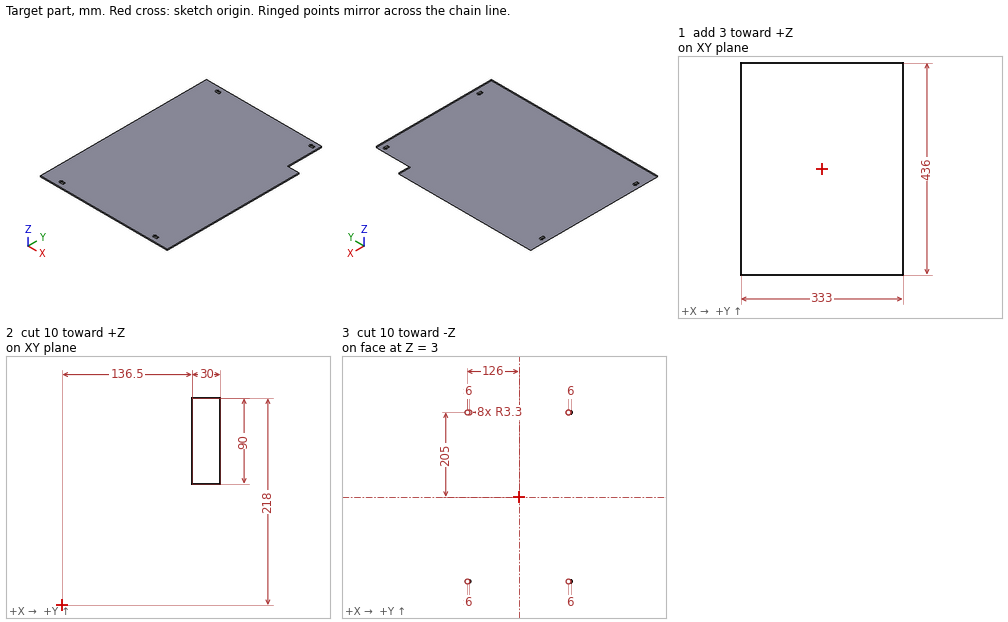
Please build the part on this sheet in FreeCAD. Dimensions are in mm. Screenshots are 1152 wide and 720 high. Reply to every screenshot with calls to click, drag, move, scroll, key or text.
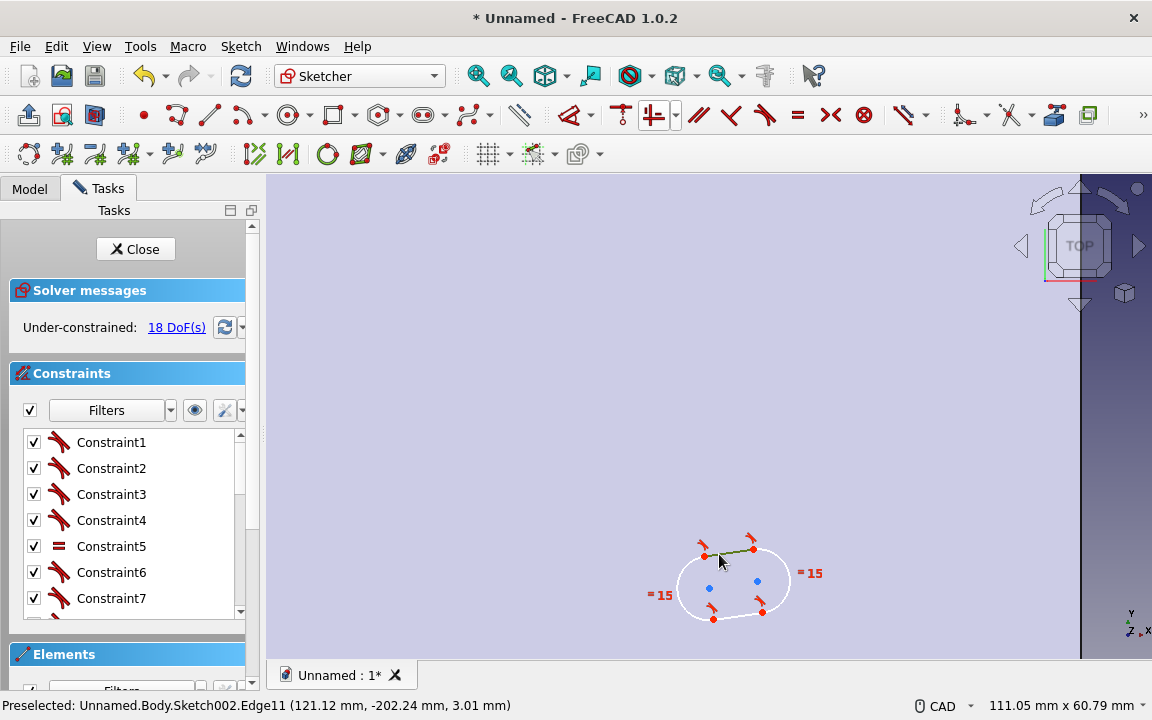
key(h)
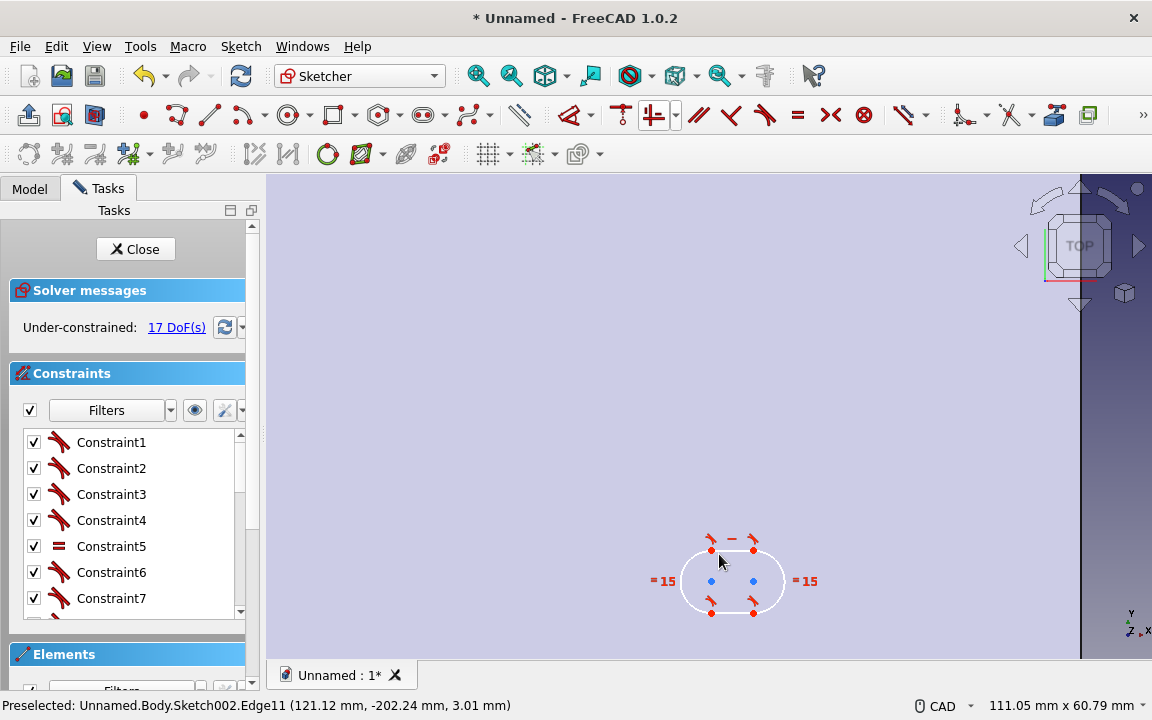
scroll(729, 564, down, 12)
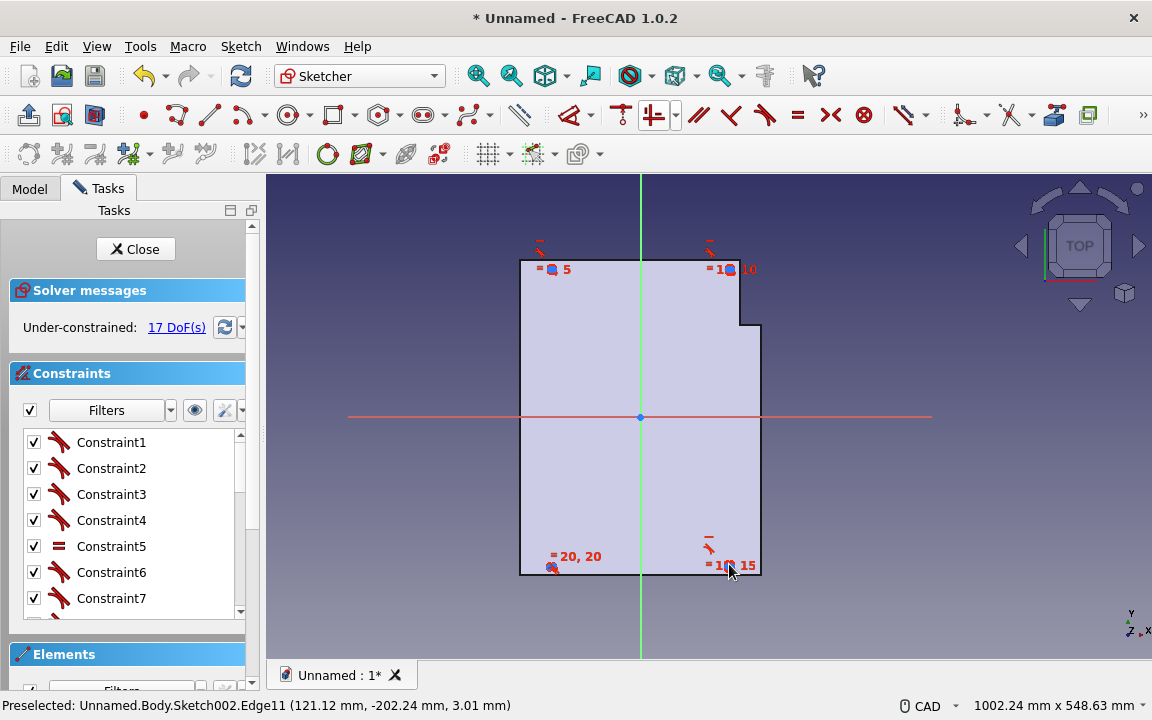
scroll(551, 566, up, 12)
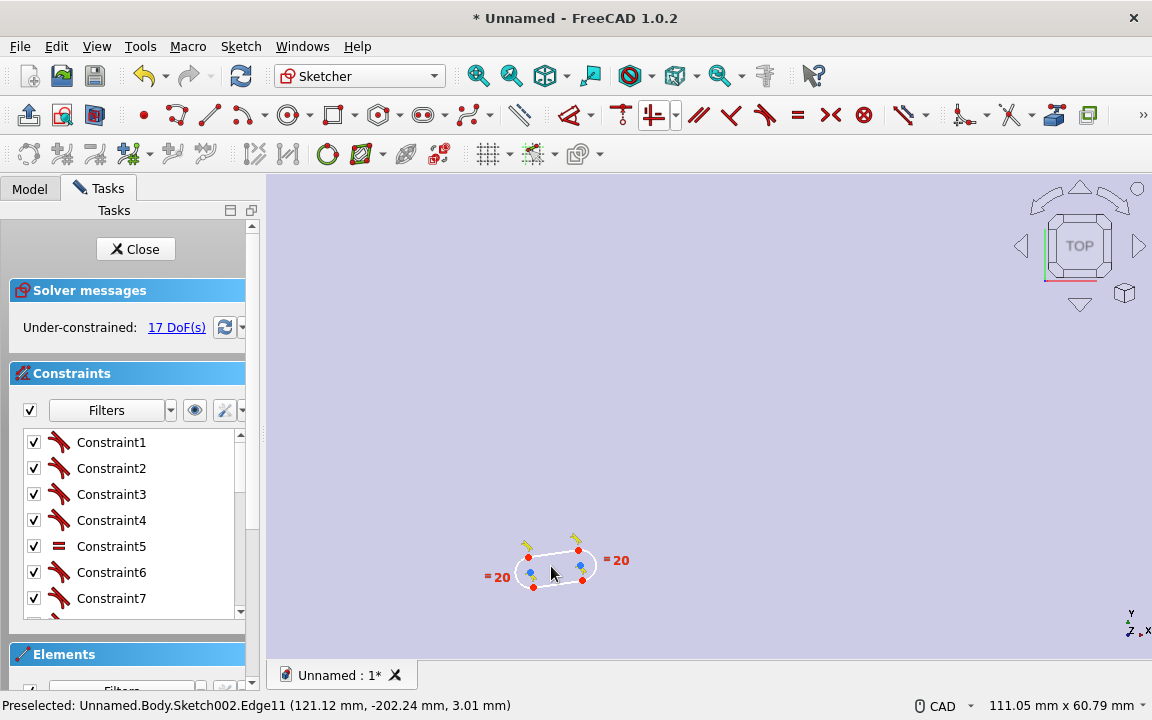
click(544, 555)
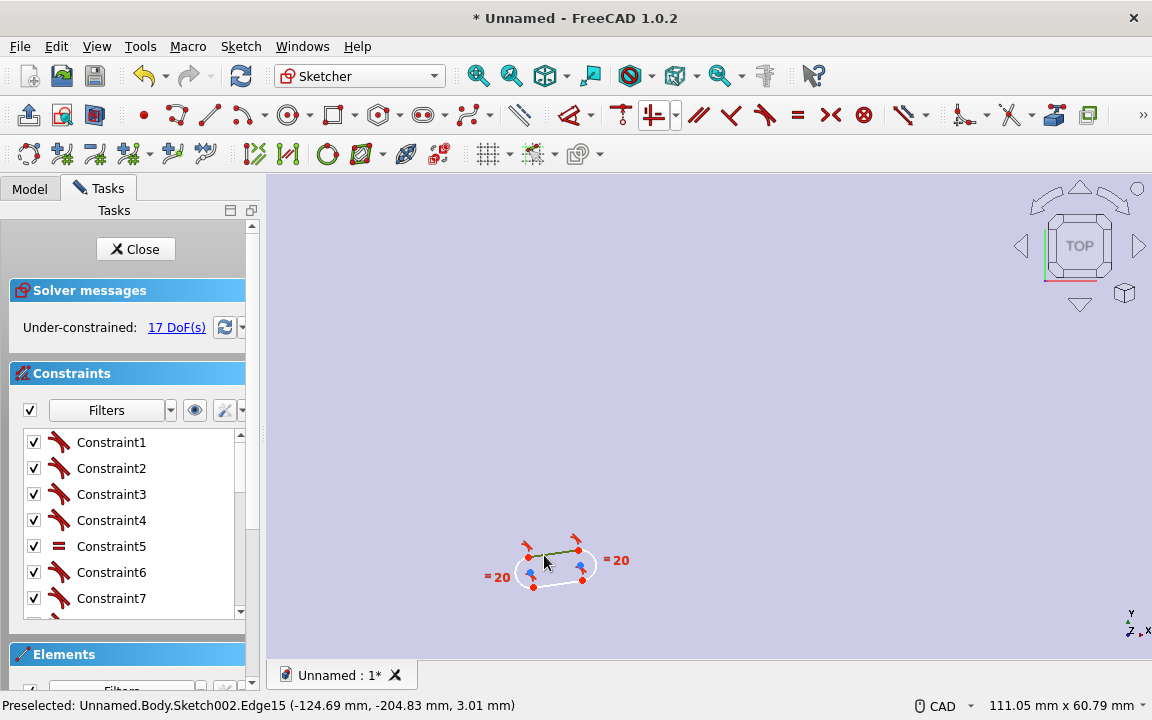
click(676, 116)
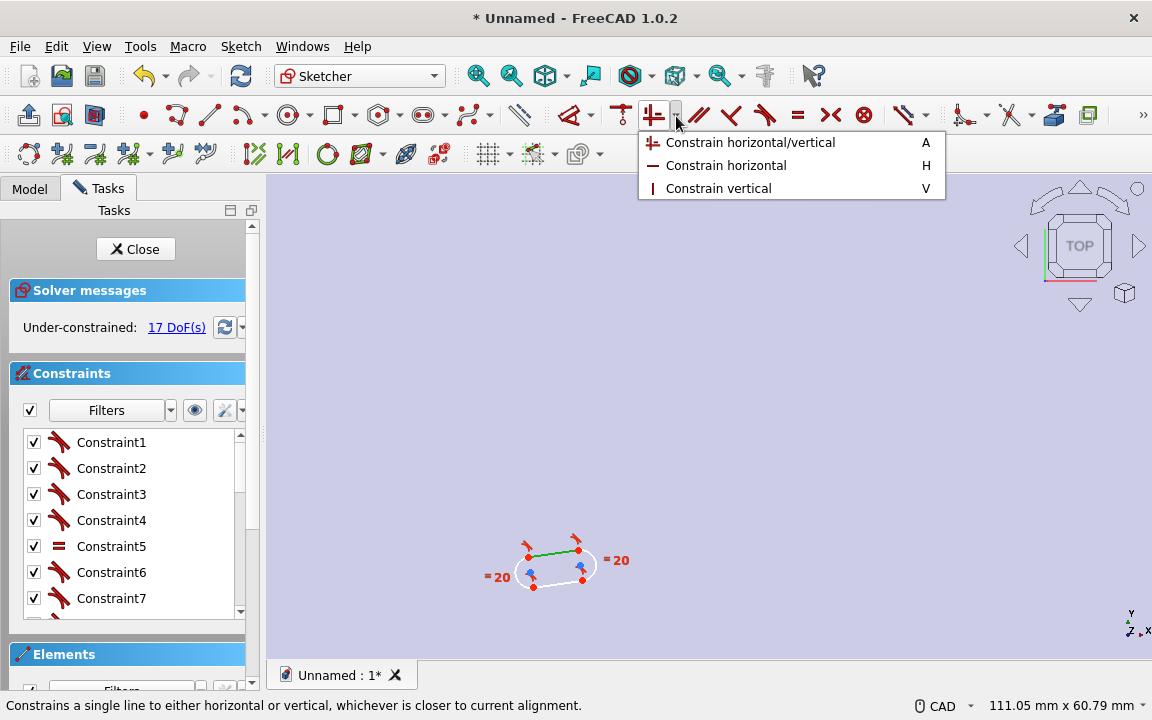
click(792, 166)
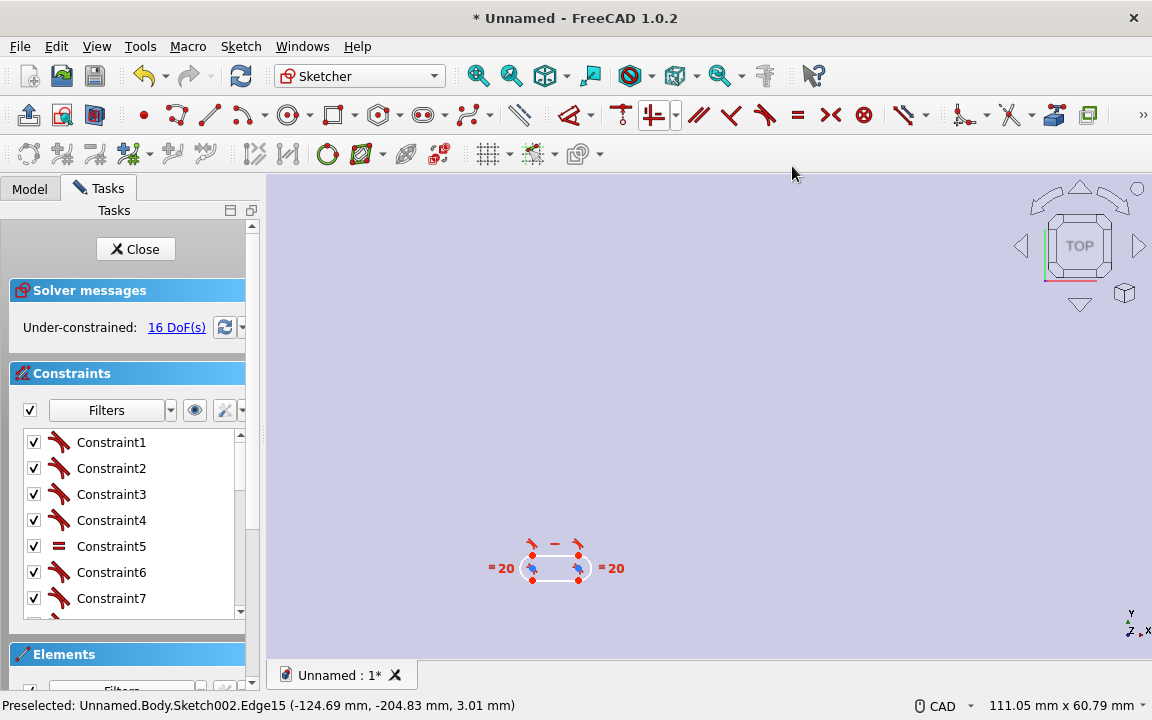
scroll(551, 566, down, 12)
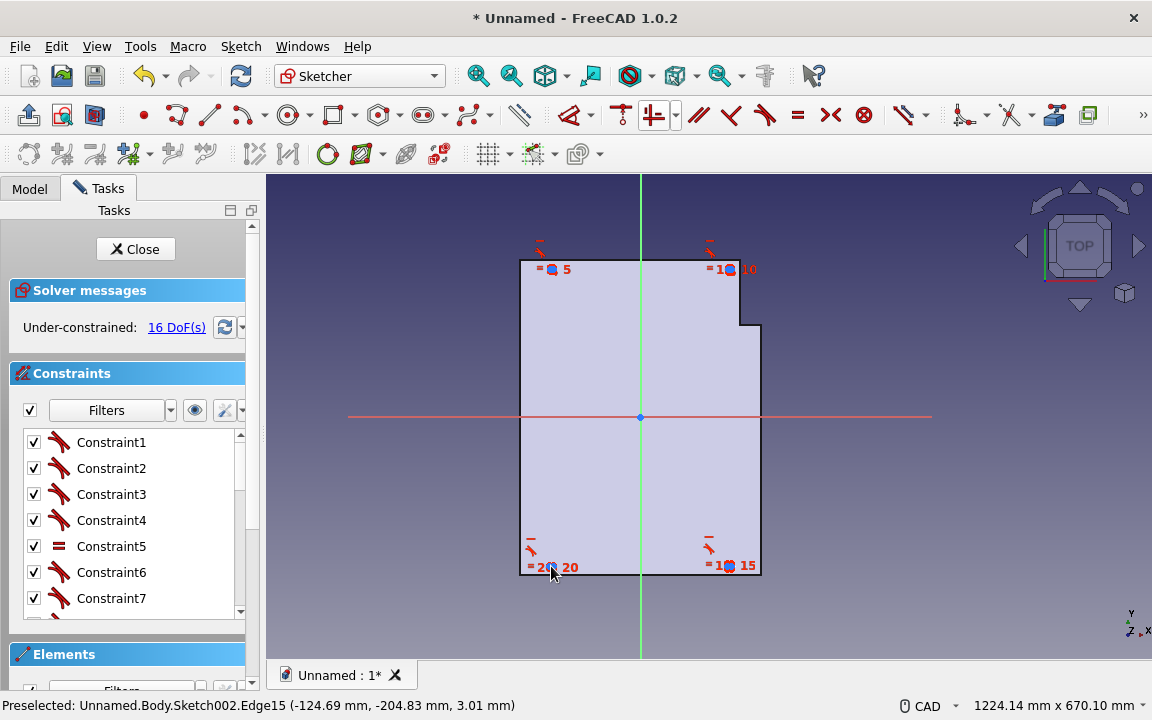
scroll(549, 268, up, 11)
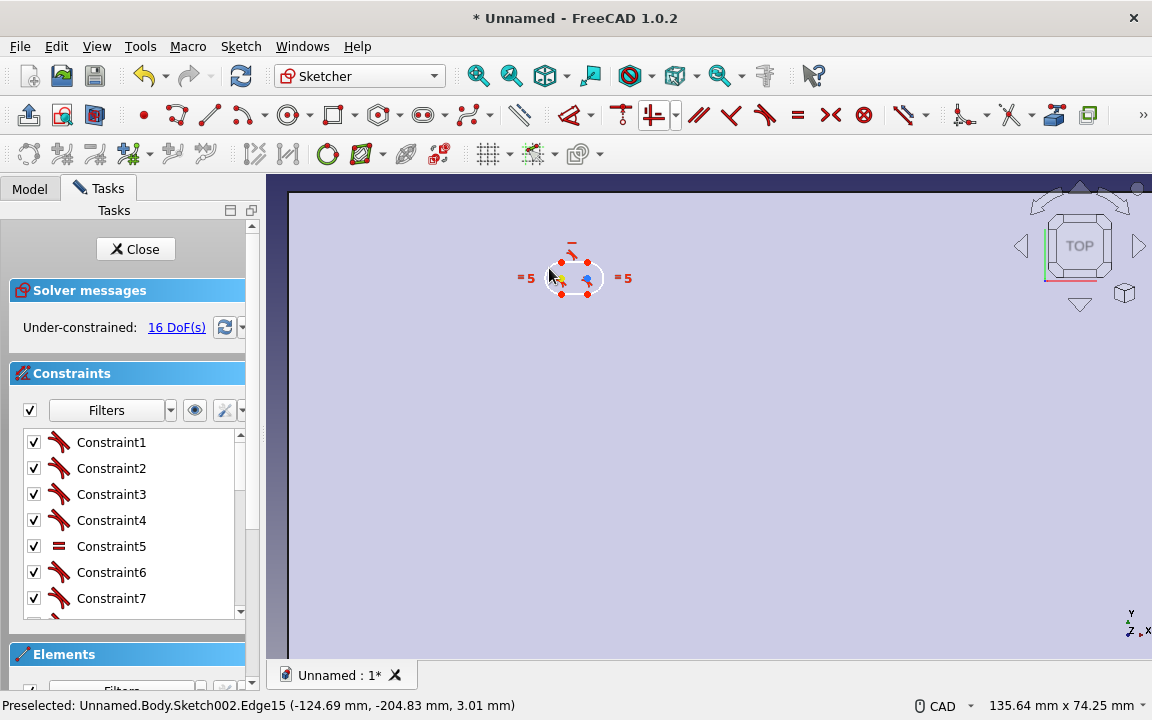
click(548, 269)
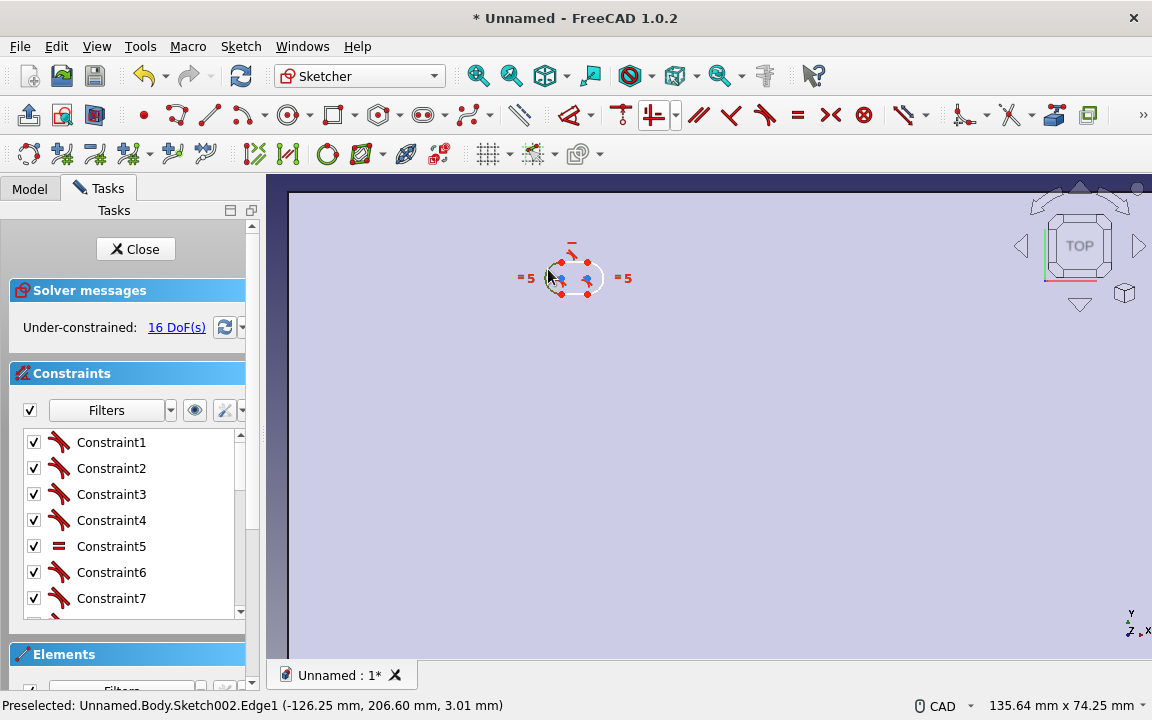
scroll(549, 267, down, 11)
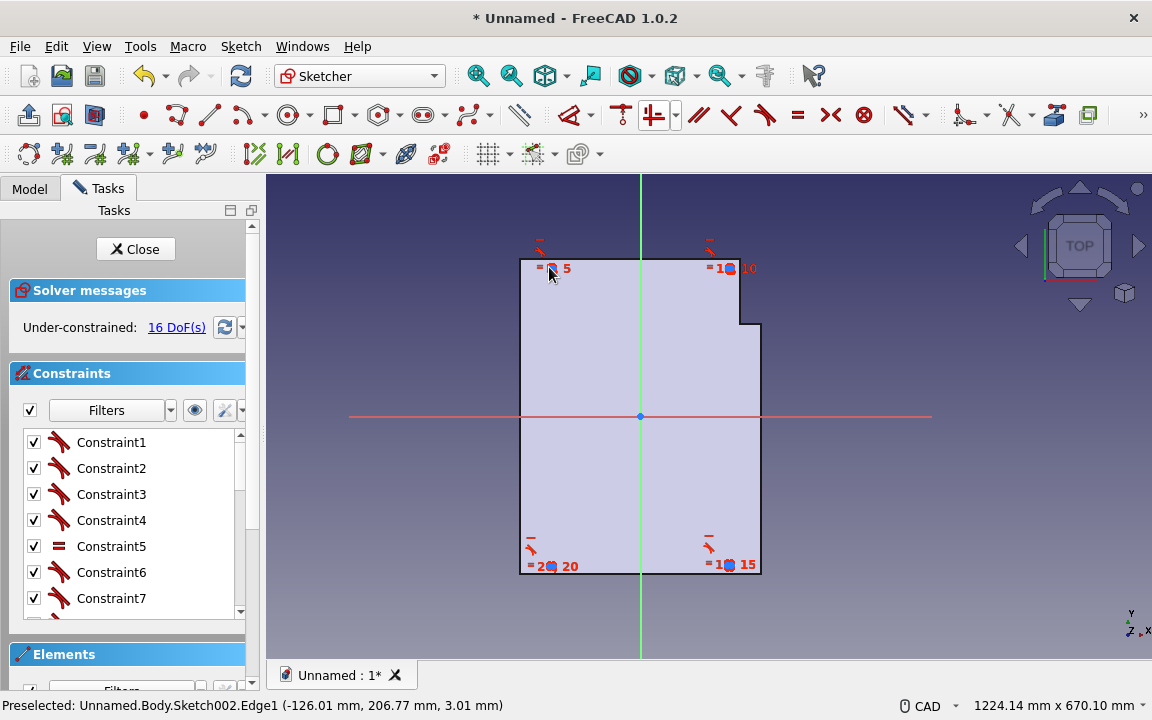
scroll(727, 267, up, 10)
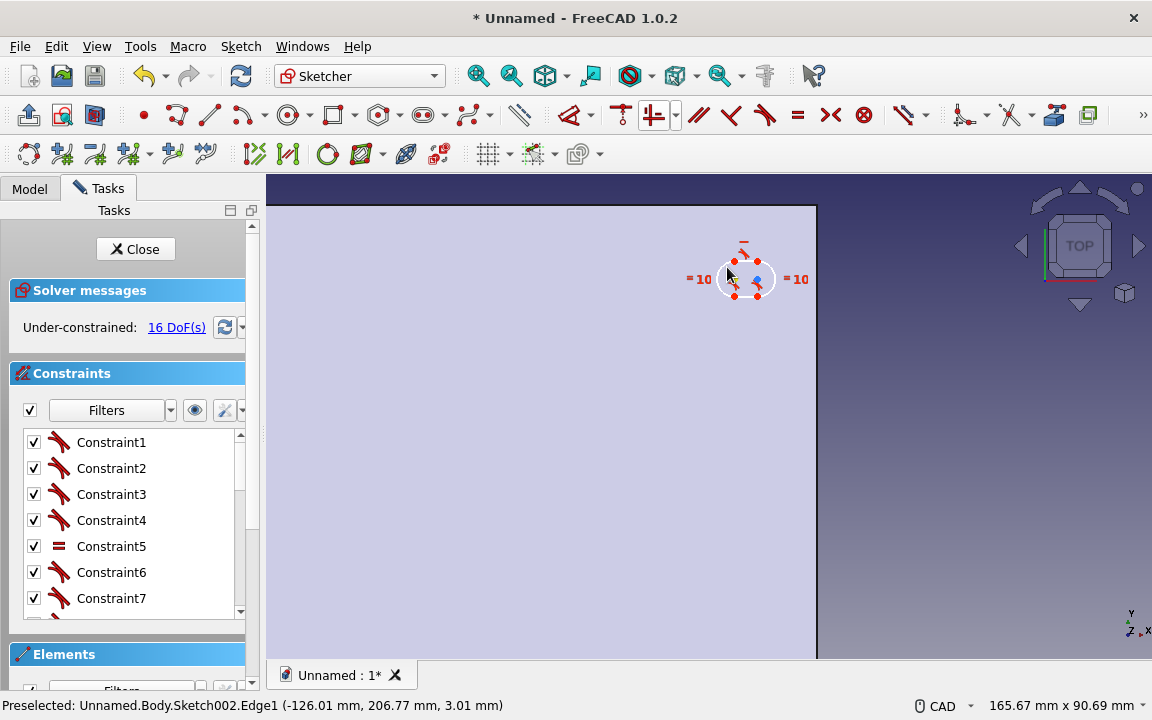
click(721, 269)